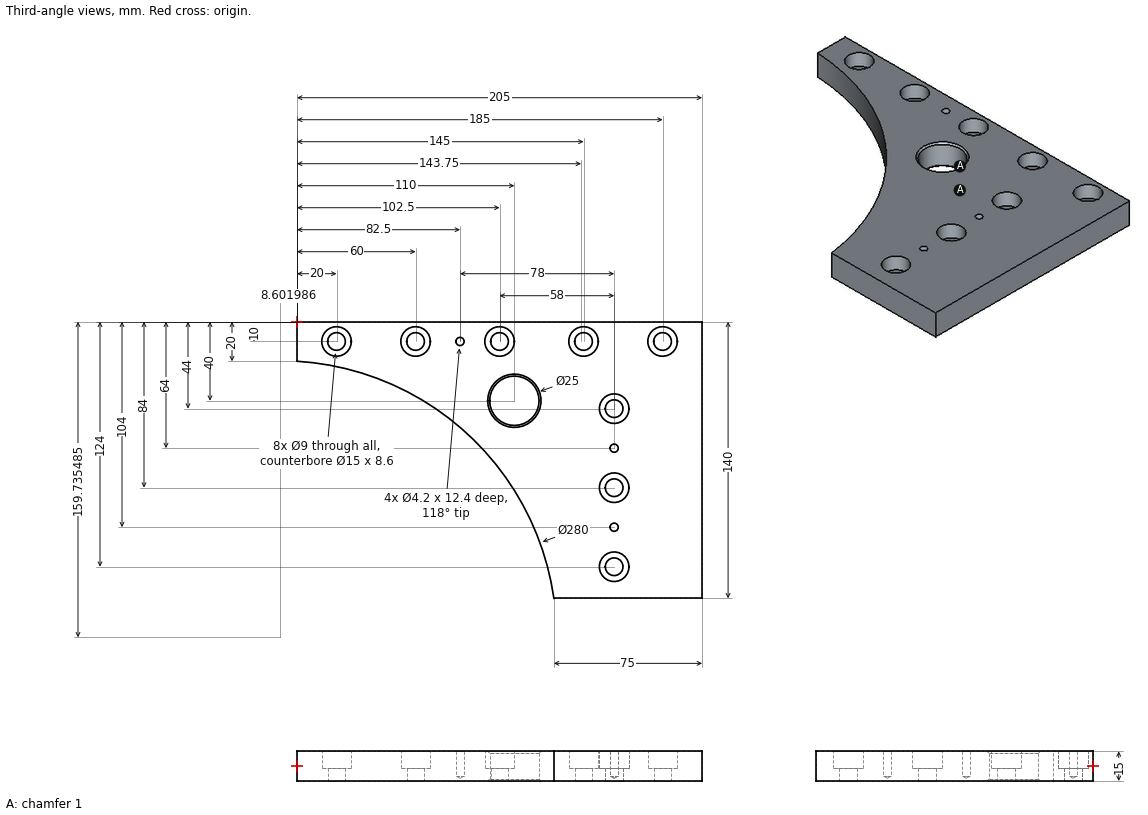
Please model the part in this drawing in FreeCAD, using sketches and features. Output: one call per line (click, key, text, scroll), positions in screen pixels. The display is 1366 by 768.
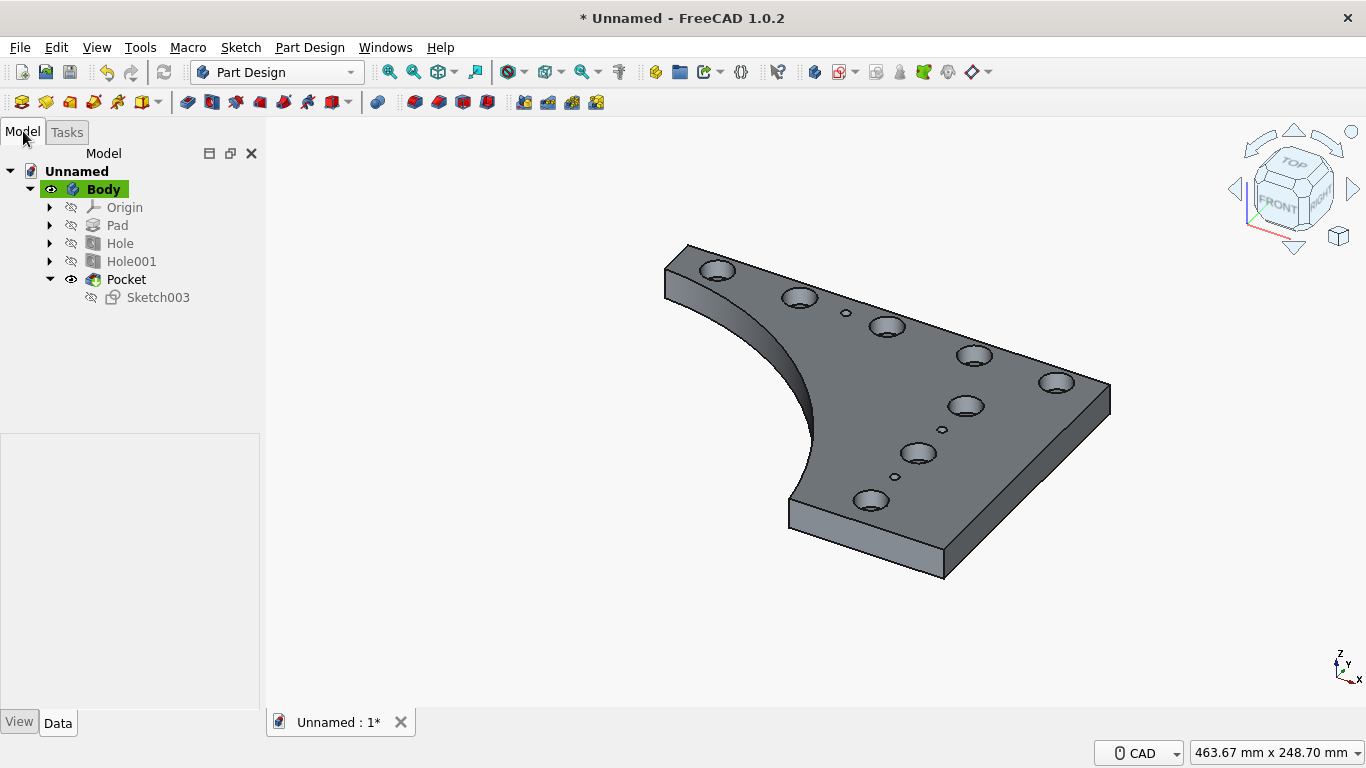
click(50, 207)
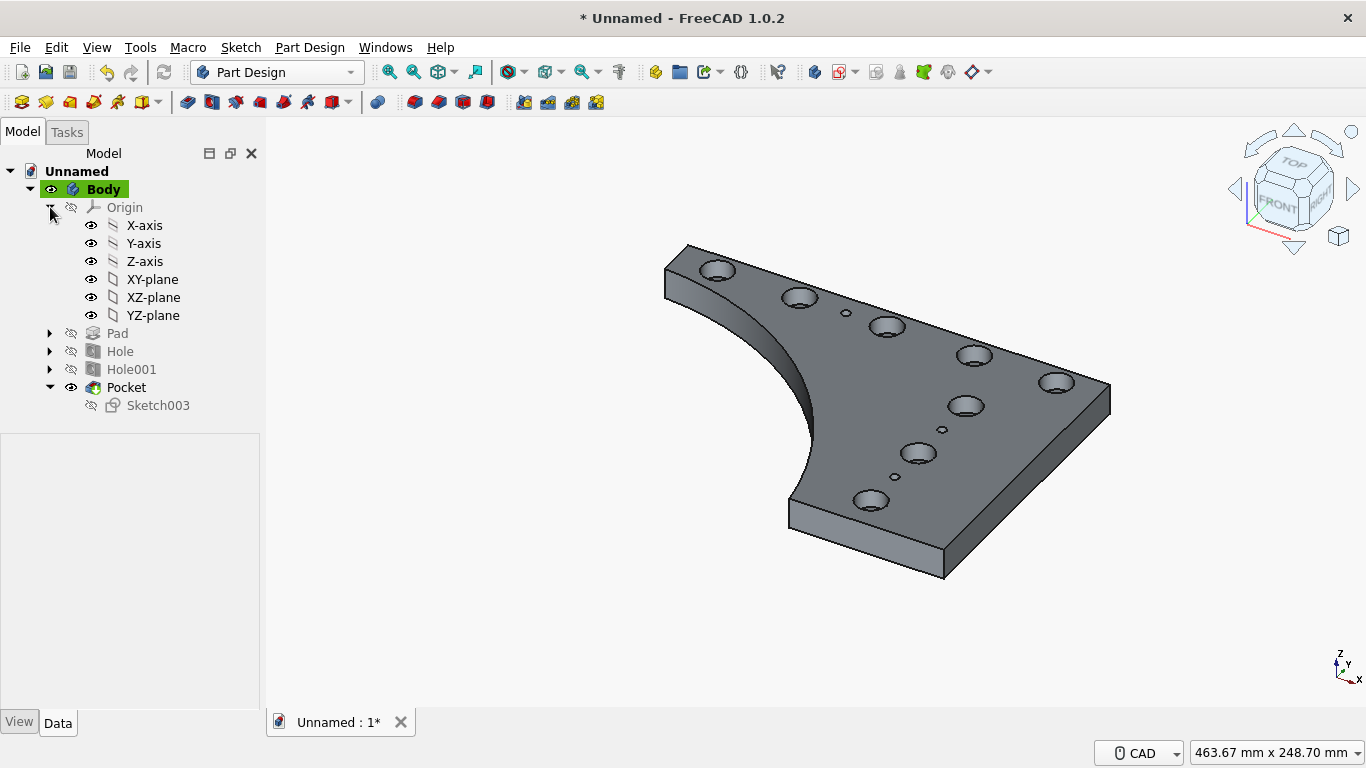
click(136, 279)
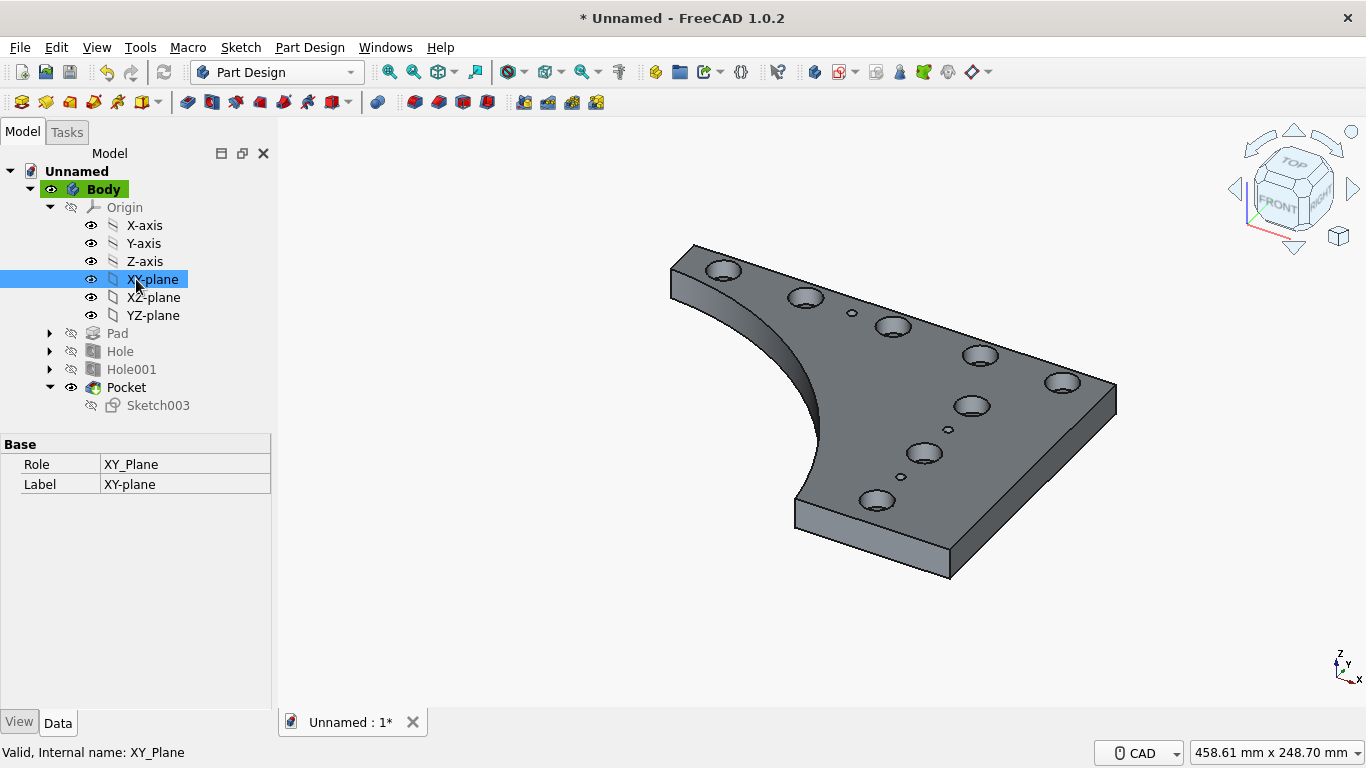
click(972, 72)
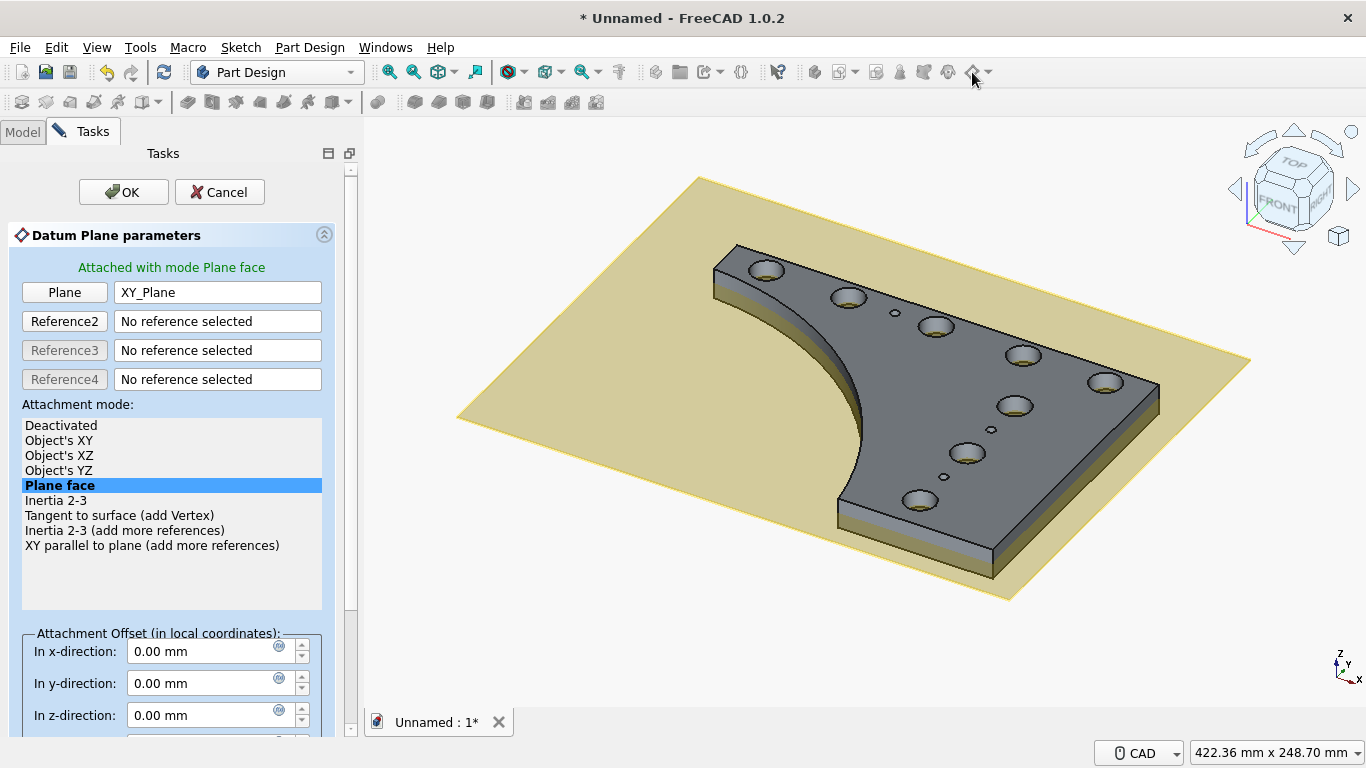
triple_click(210, 715)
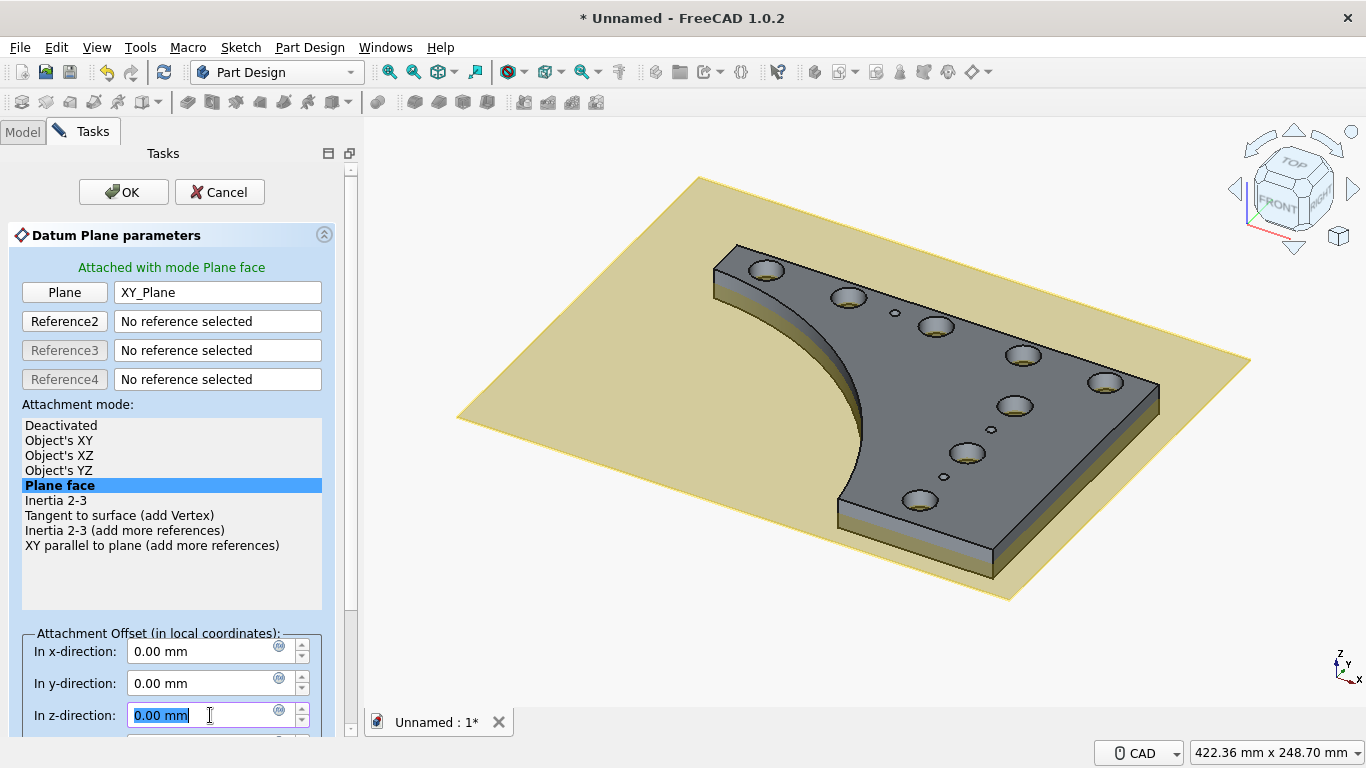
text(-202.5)
key(Tab)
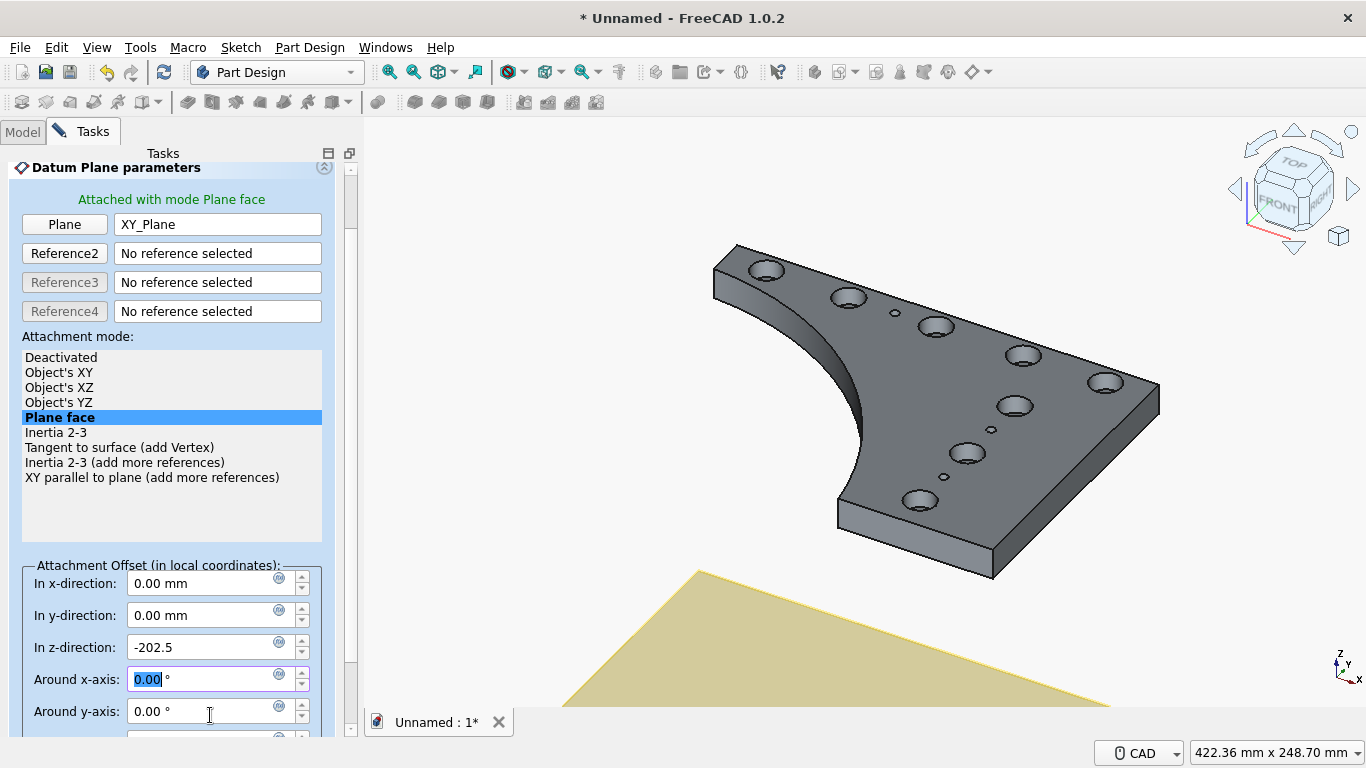
scroll(351, 450, up, 2)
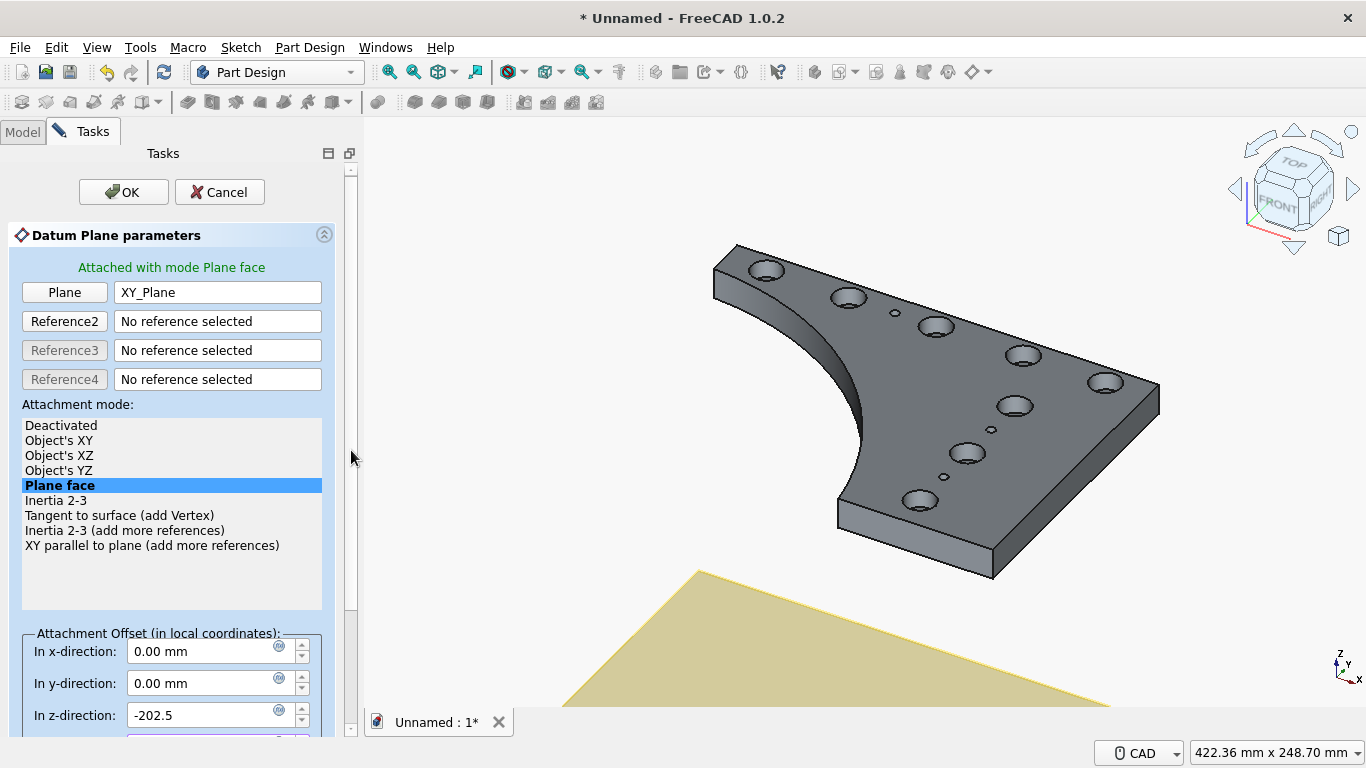
click(124, 192)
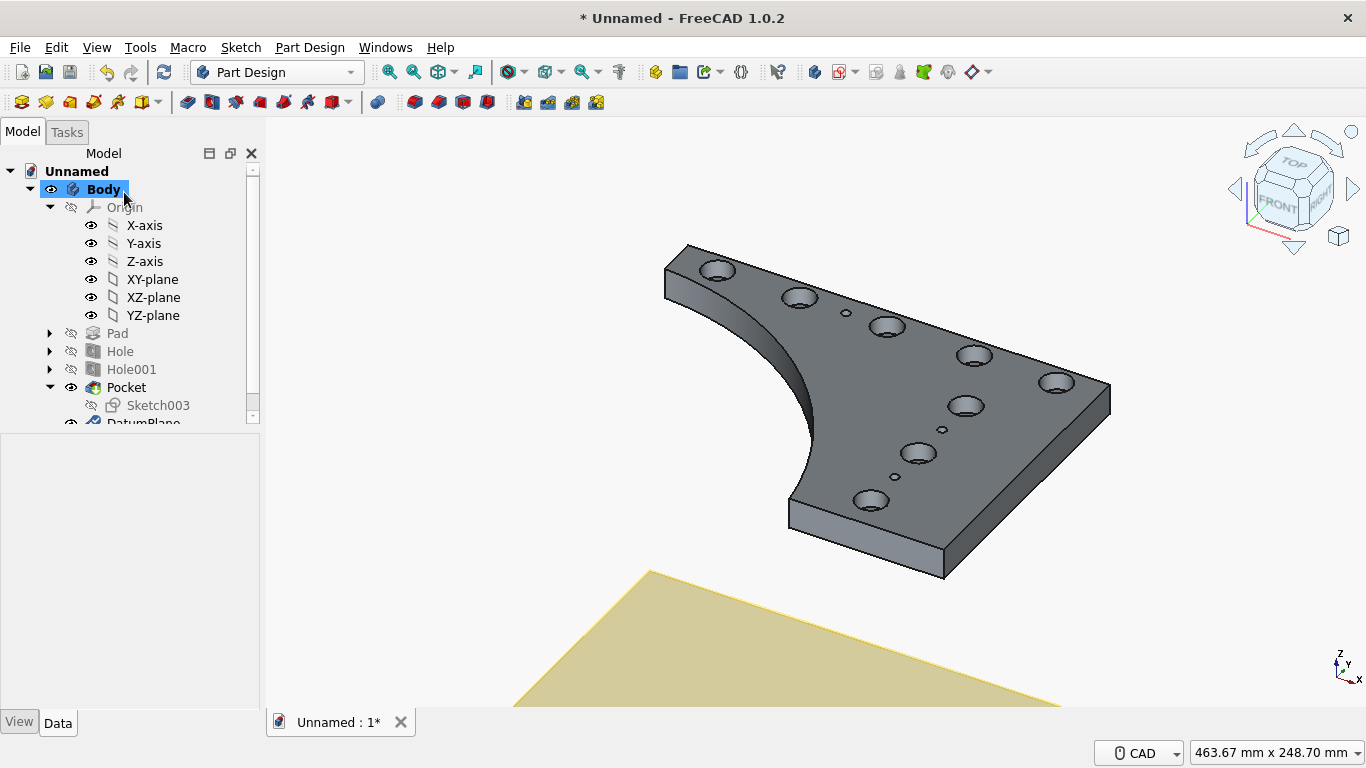
click(116, 423)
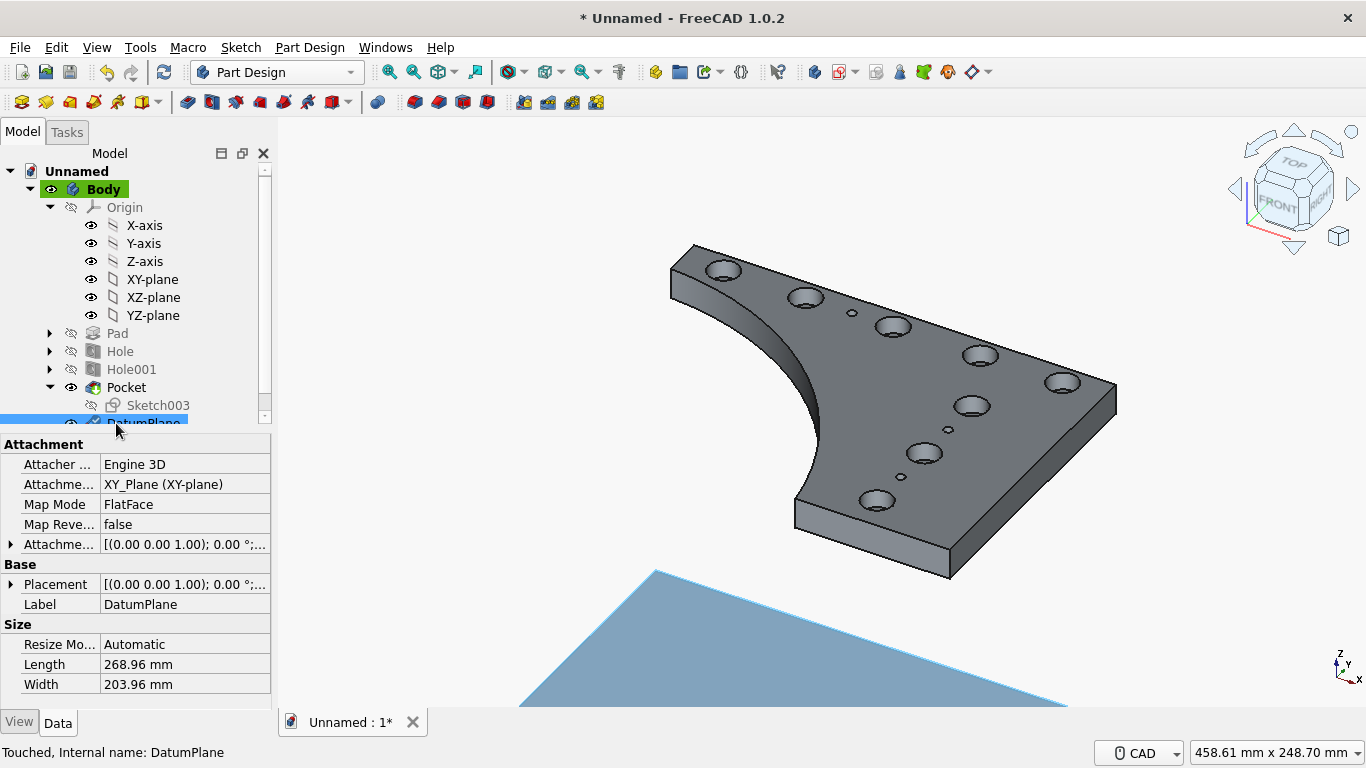
click(840, 72)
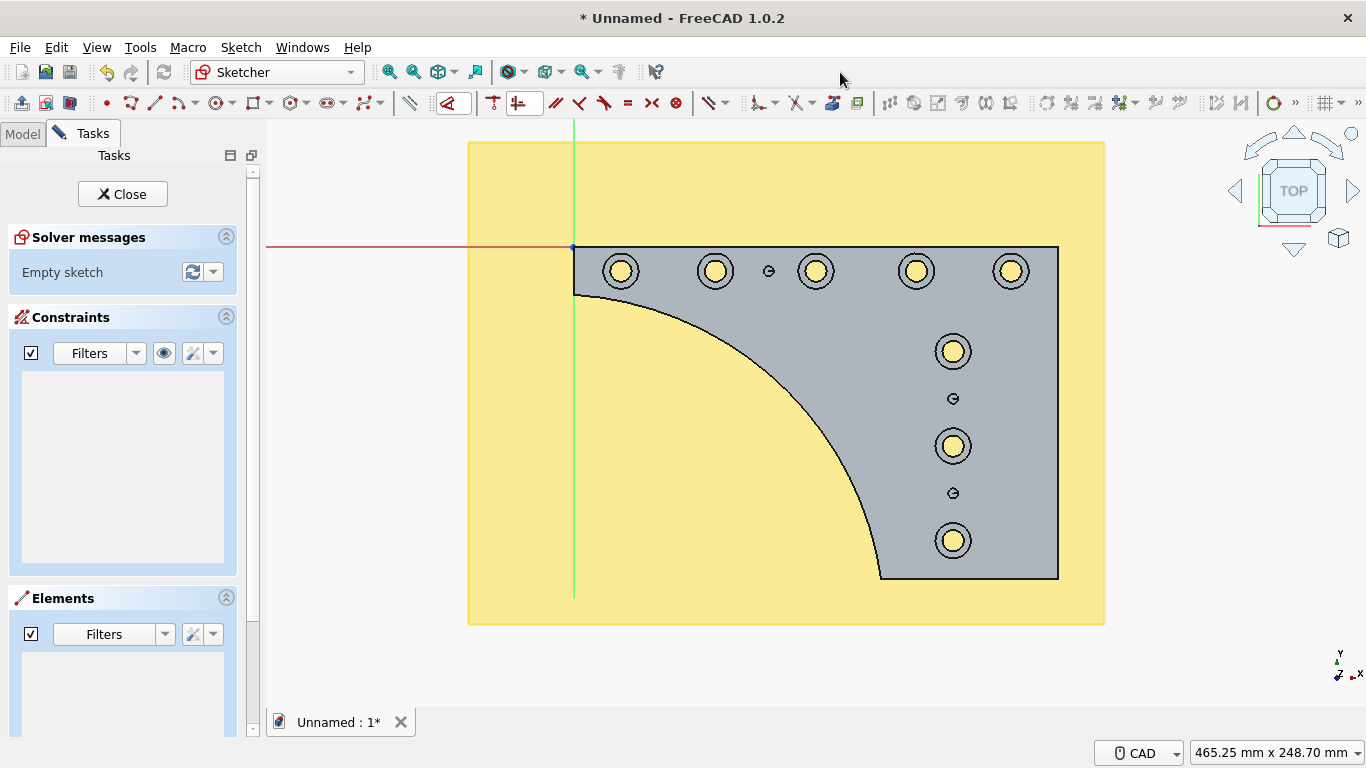
click(70, 104)